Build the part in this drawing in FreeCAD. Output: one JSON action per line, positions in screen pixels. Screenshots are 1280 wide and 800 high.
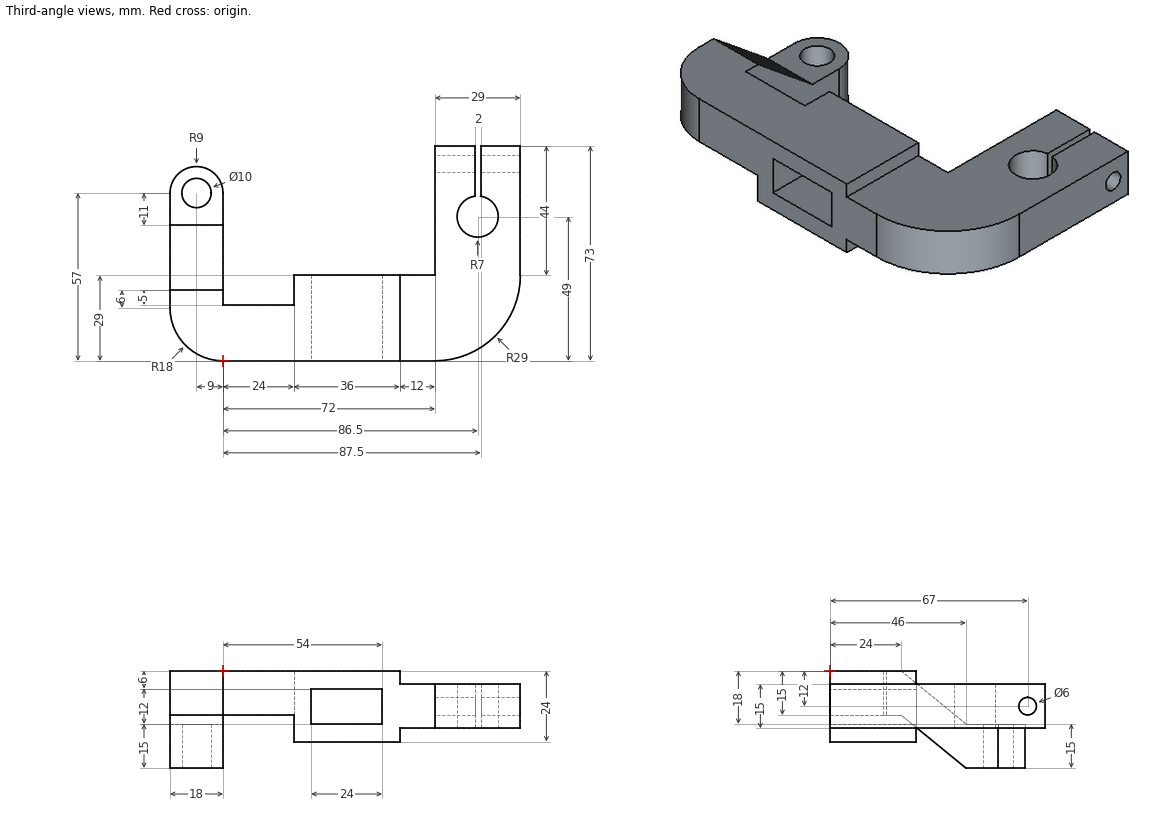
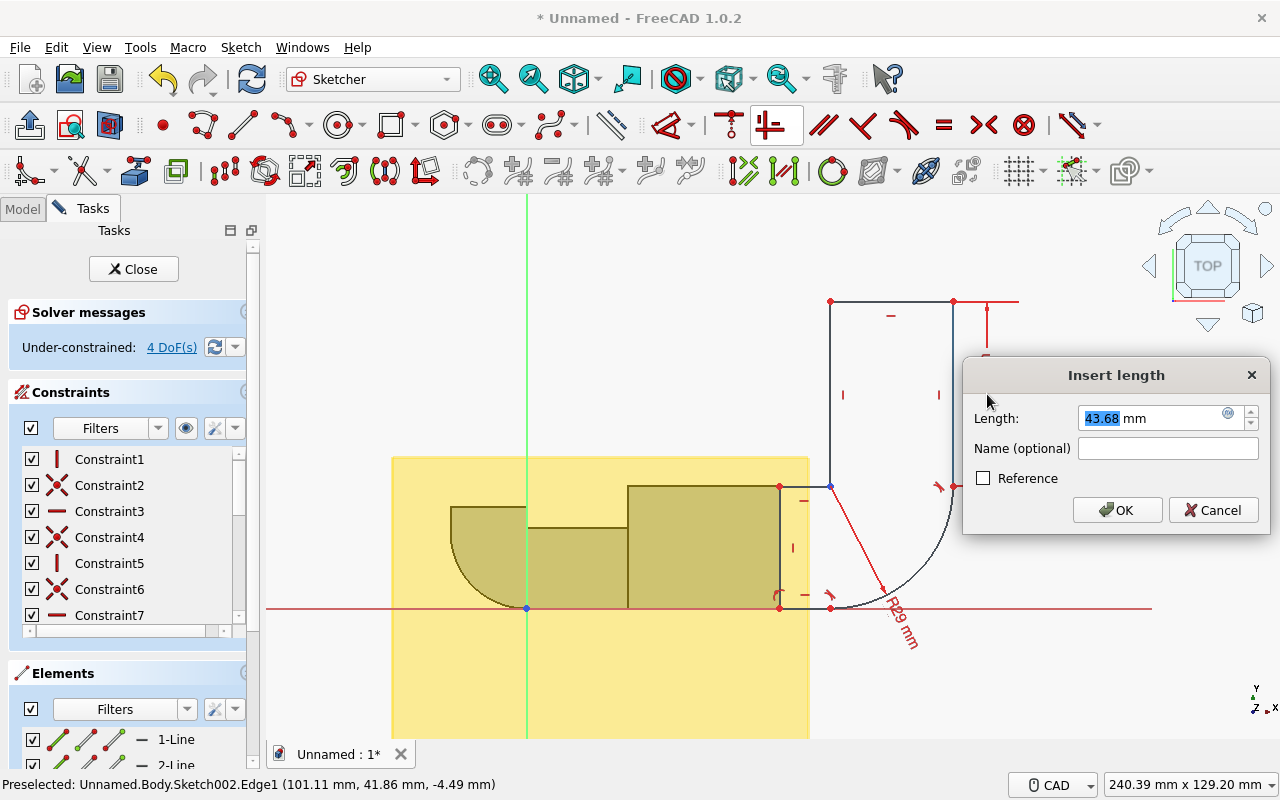
{"action": "type", "text": "44"}
{"action": "key", "text": "Return"}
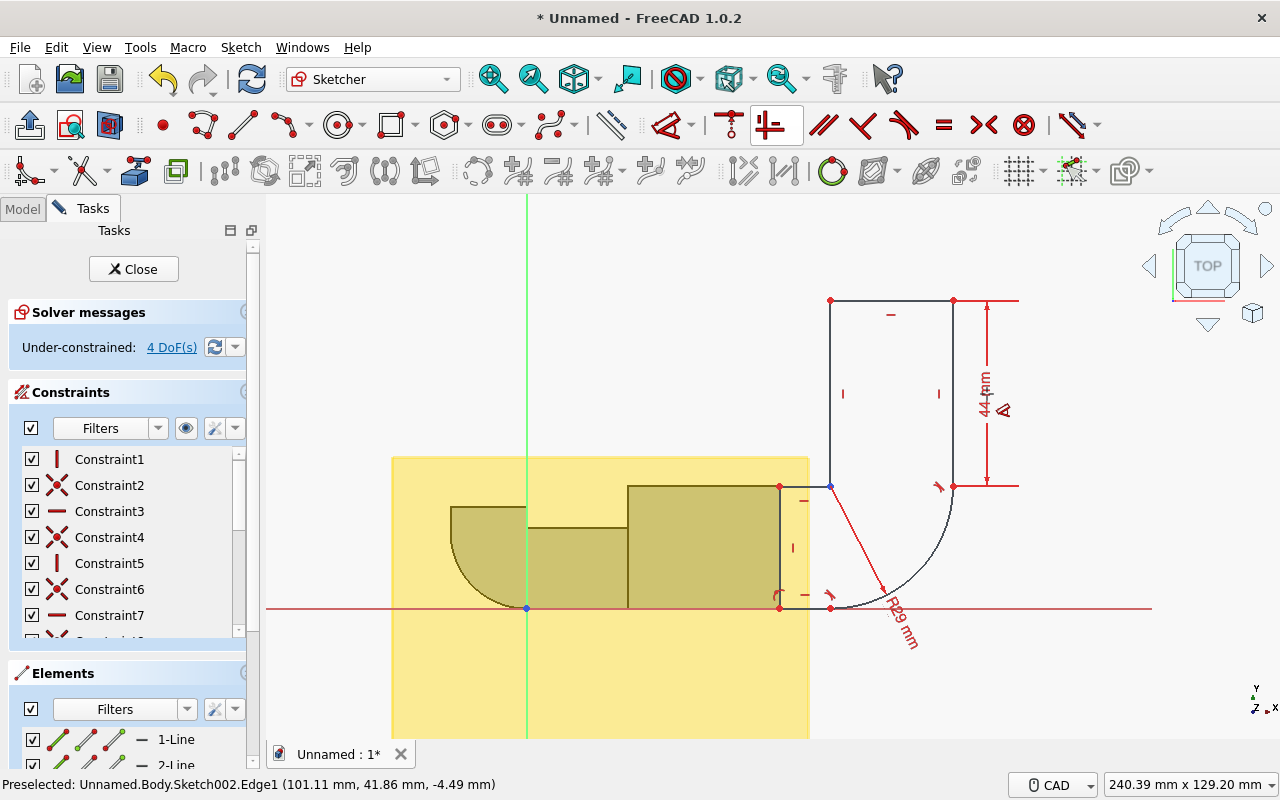
{"action": "left_click", "coordinate": [916, 301]}
{"action": "left_click", "coordinate": [892, 267]}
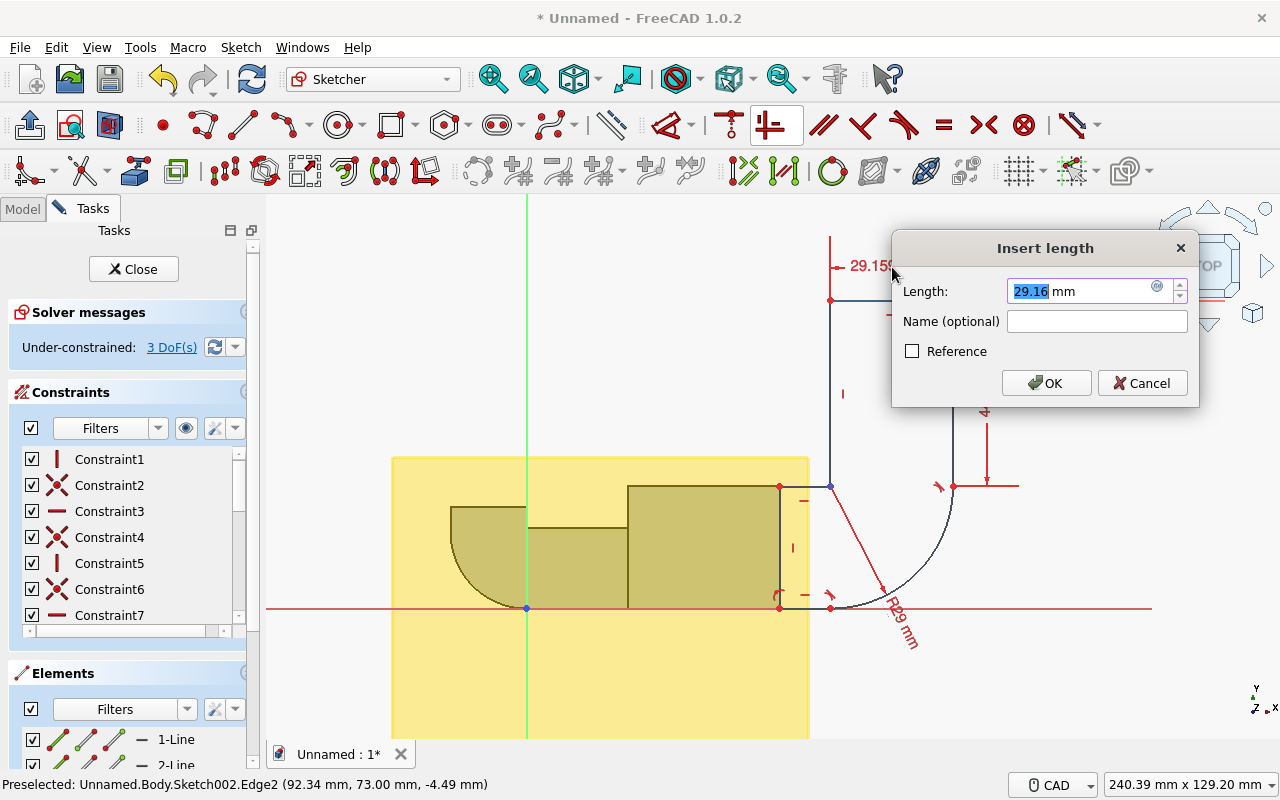
{"action": "type", "text": "29"}
{"action": "key", "text": "Return"}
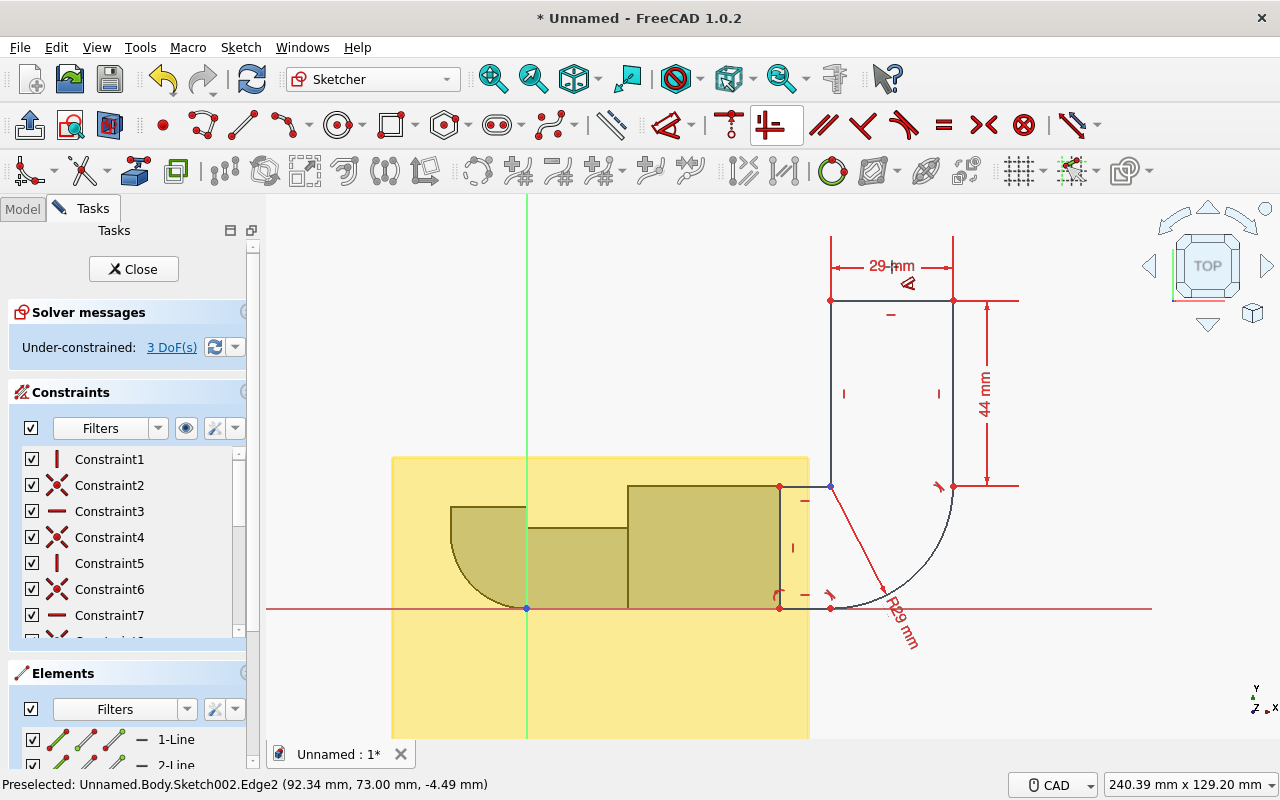
{"action": "left_click", "coordinate": [831, 357]}
{"action": "left_click", "coordinate": [865, 394]}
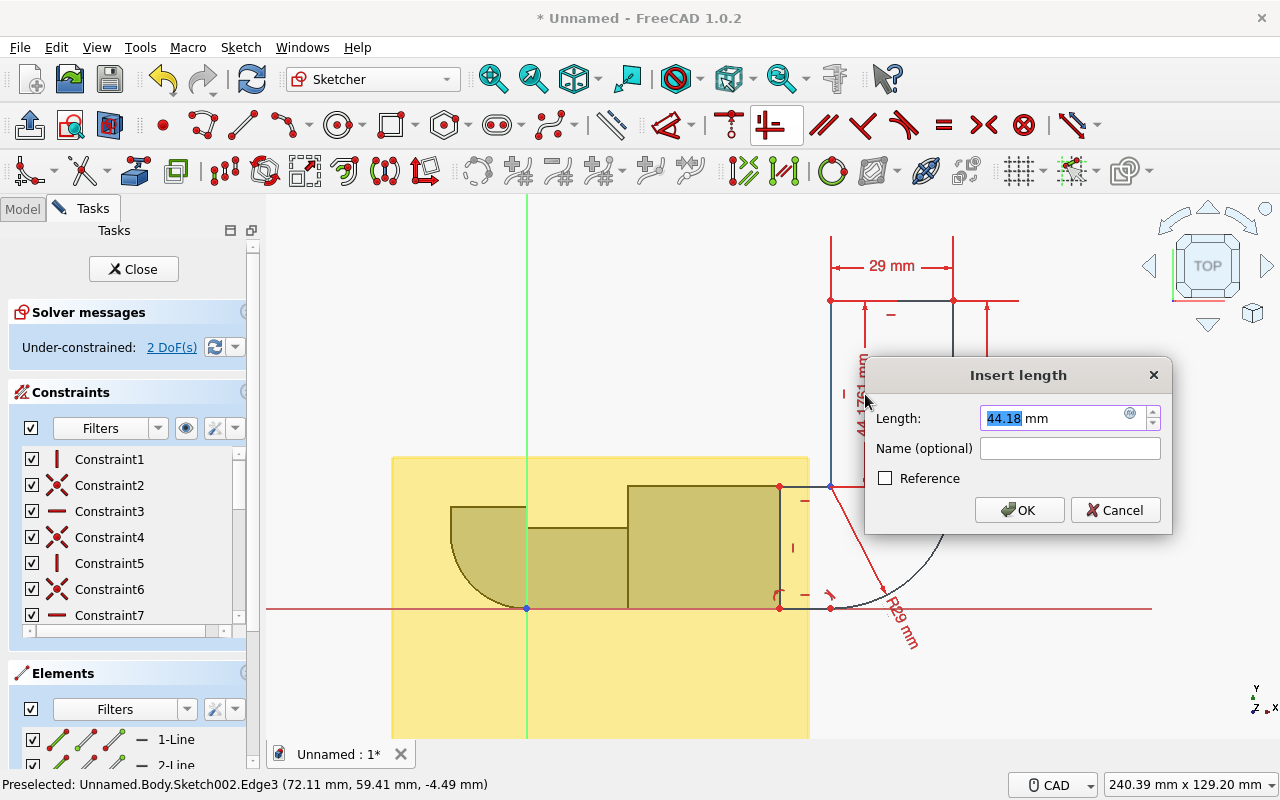
{"action": "type", "text": "44"}
{"action": "key", "text": "Return"}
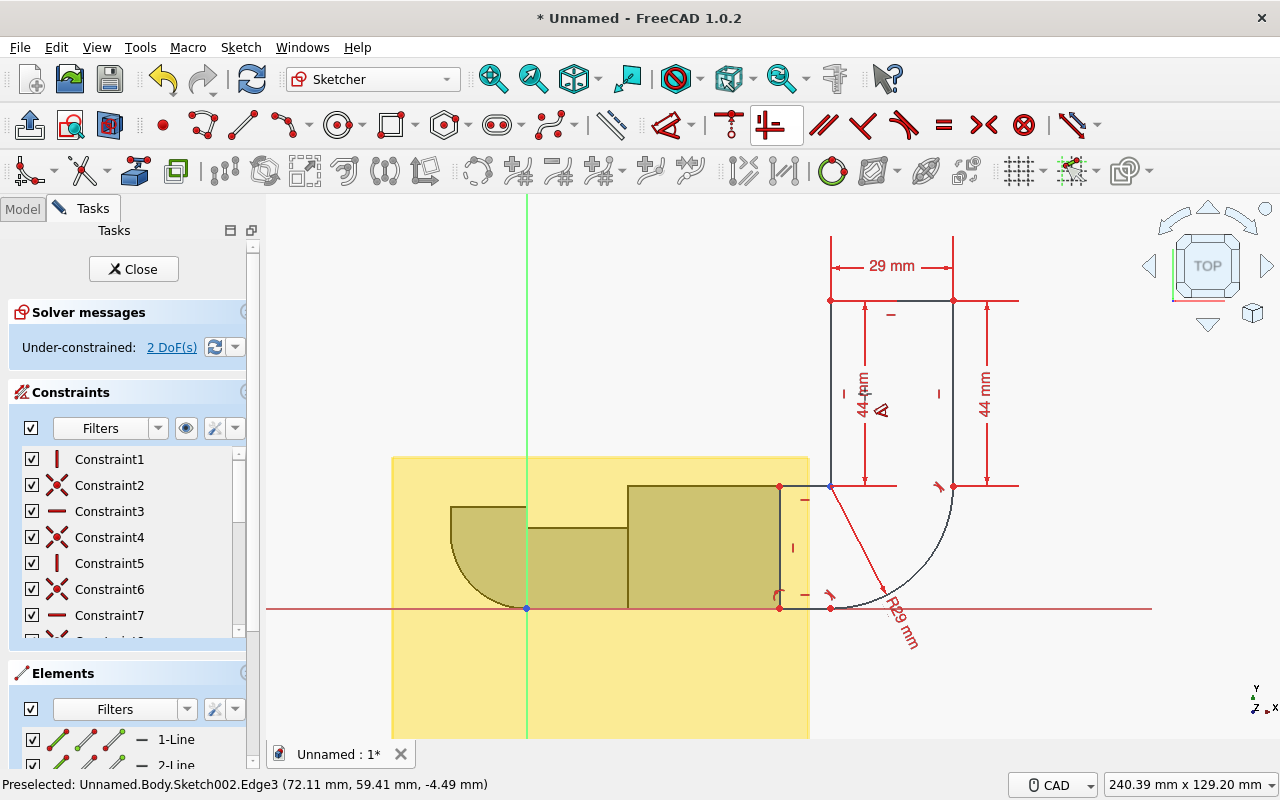
{"action": "left_click", "coordinate": [815, 486]}
{"action": "left_click", "coordinate": [805, 520]}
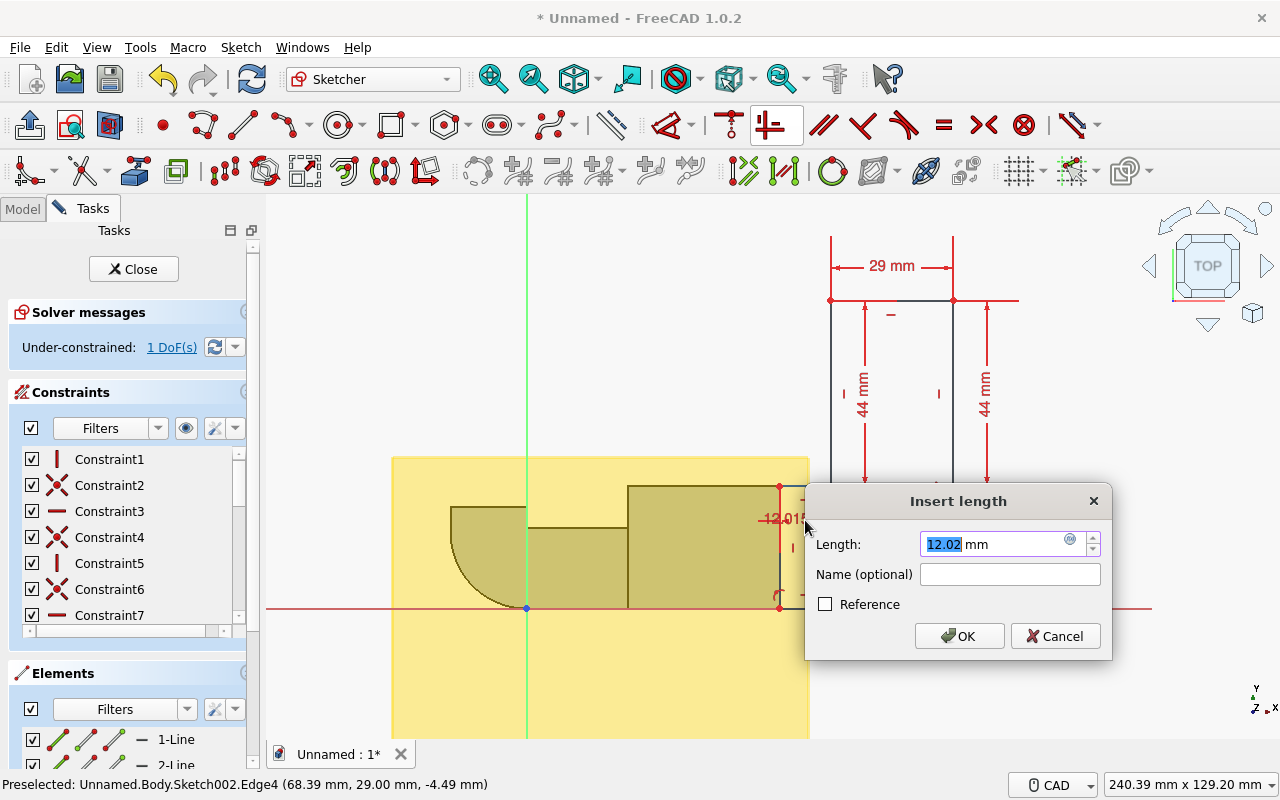
{"action": "type", "text": "12"}
{"action": "key", "text": "Return"}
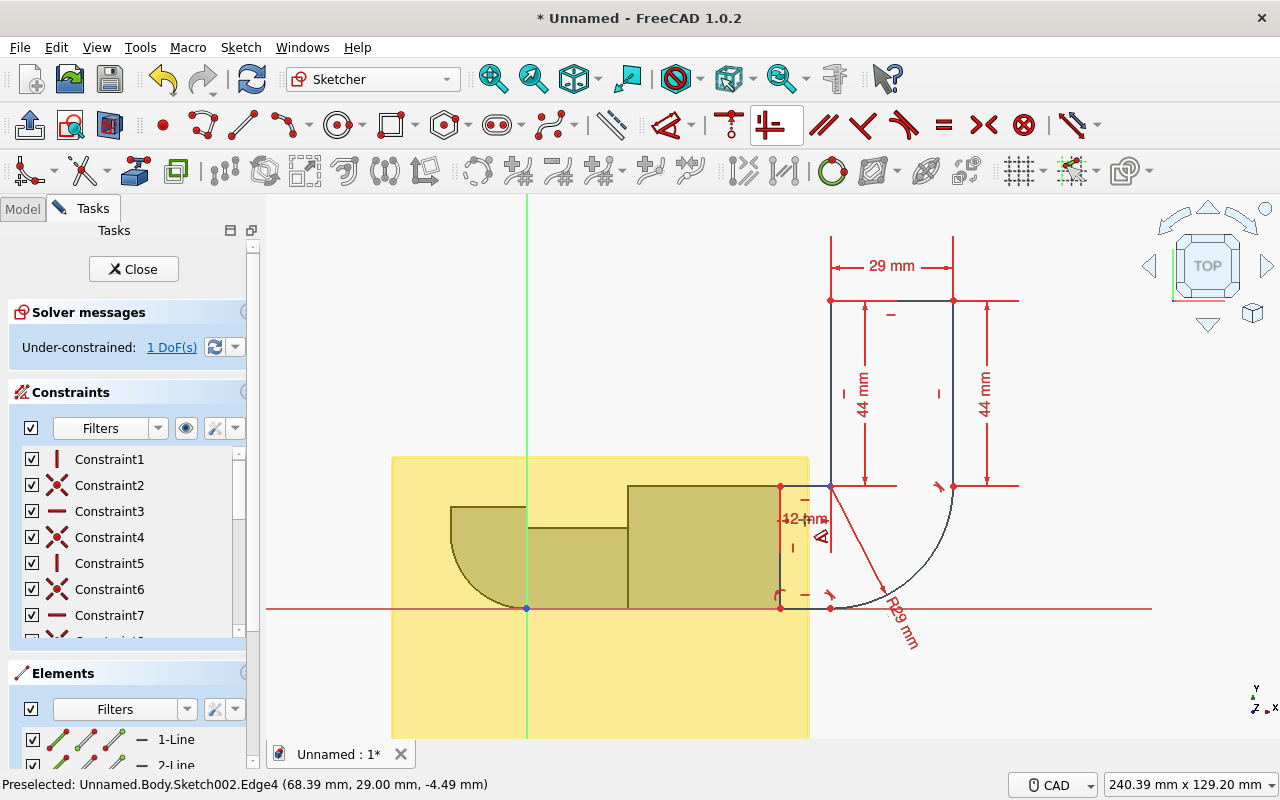
{"action": "left_click", "coordinate": [831, 301]}
{"action": "left_click", "coordinate": [679, 643]}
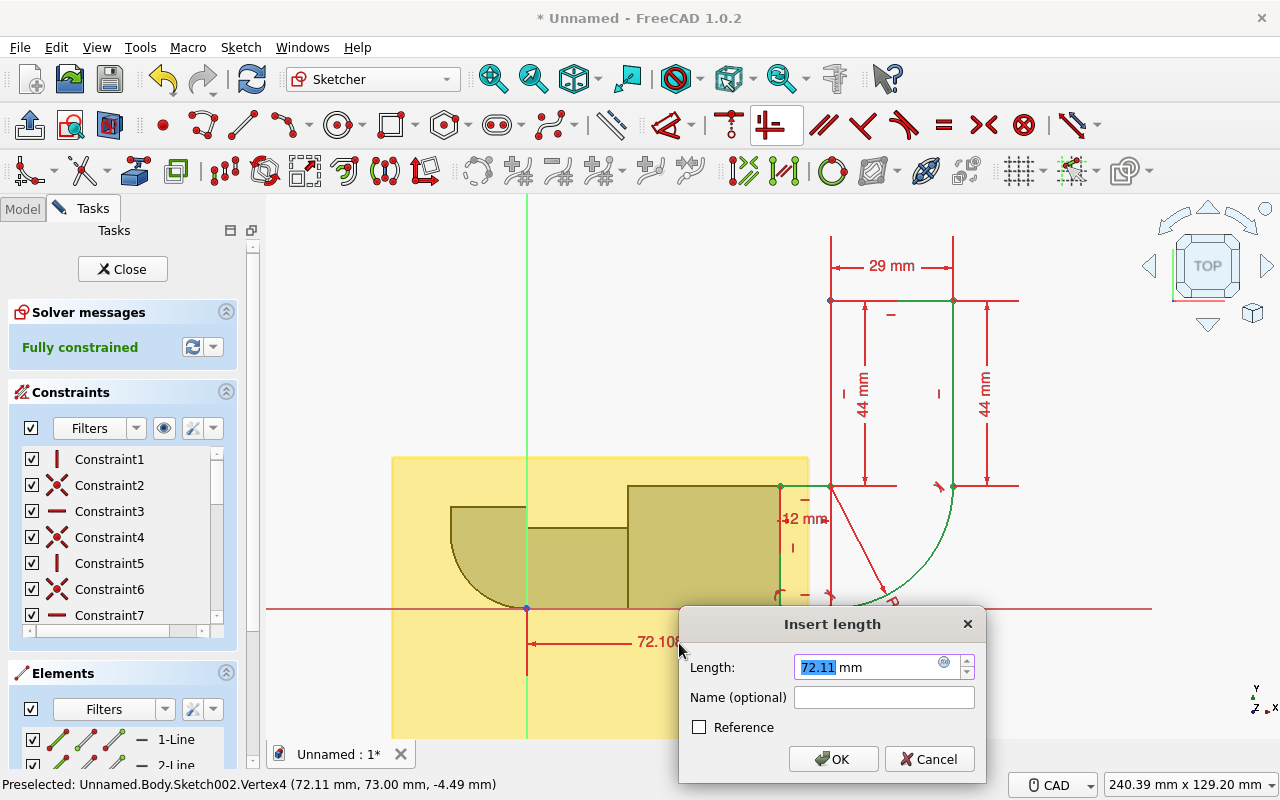
{"action": "type", "text": "72"}
{"action": "key", "text": "Return"}
{"action": "key", "text": "Escape"}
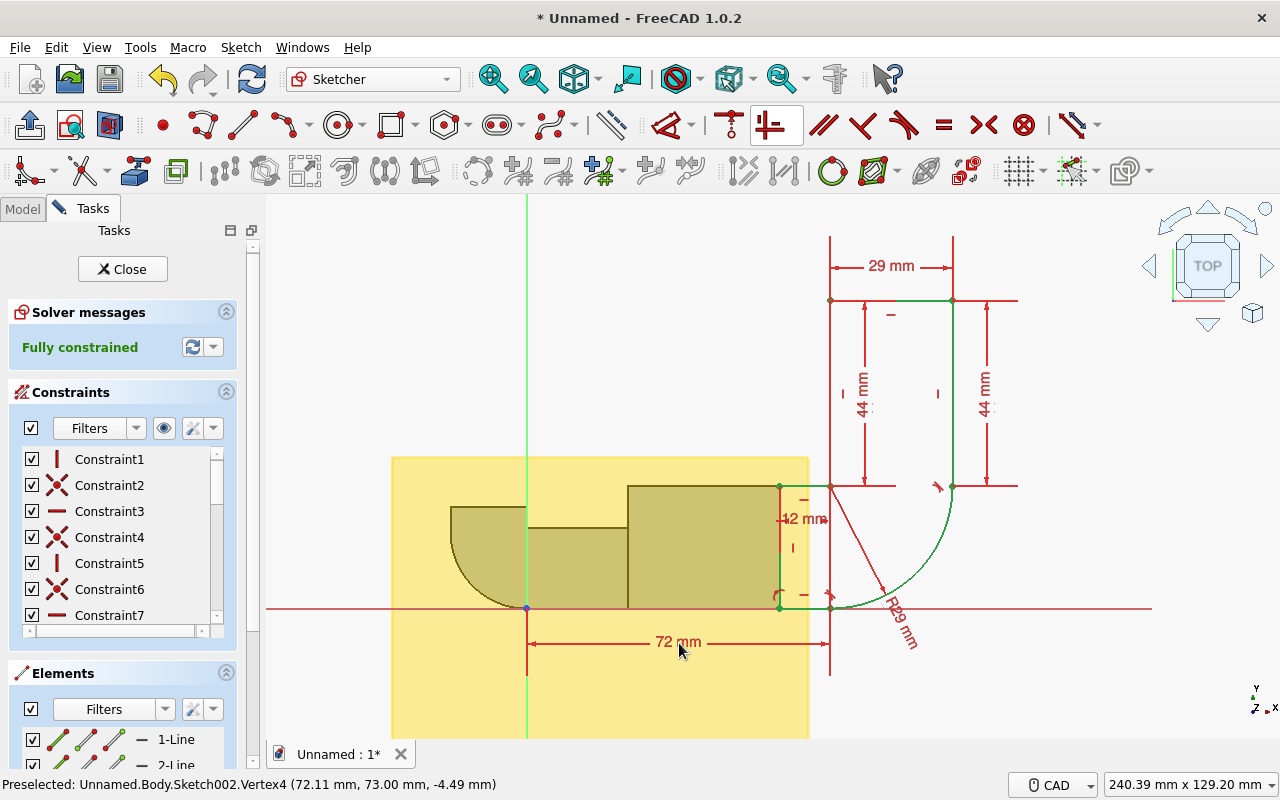
{"action": "left_click", "coordinate": [123, 269]}